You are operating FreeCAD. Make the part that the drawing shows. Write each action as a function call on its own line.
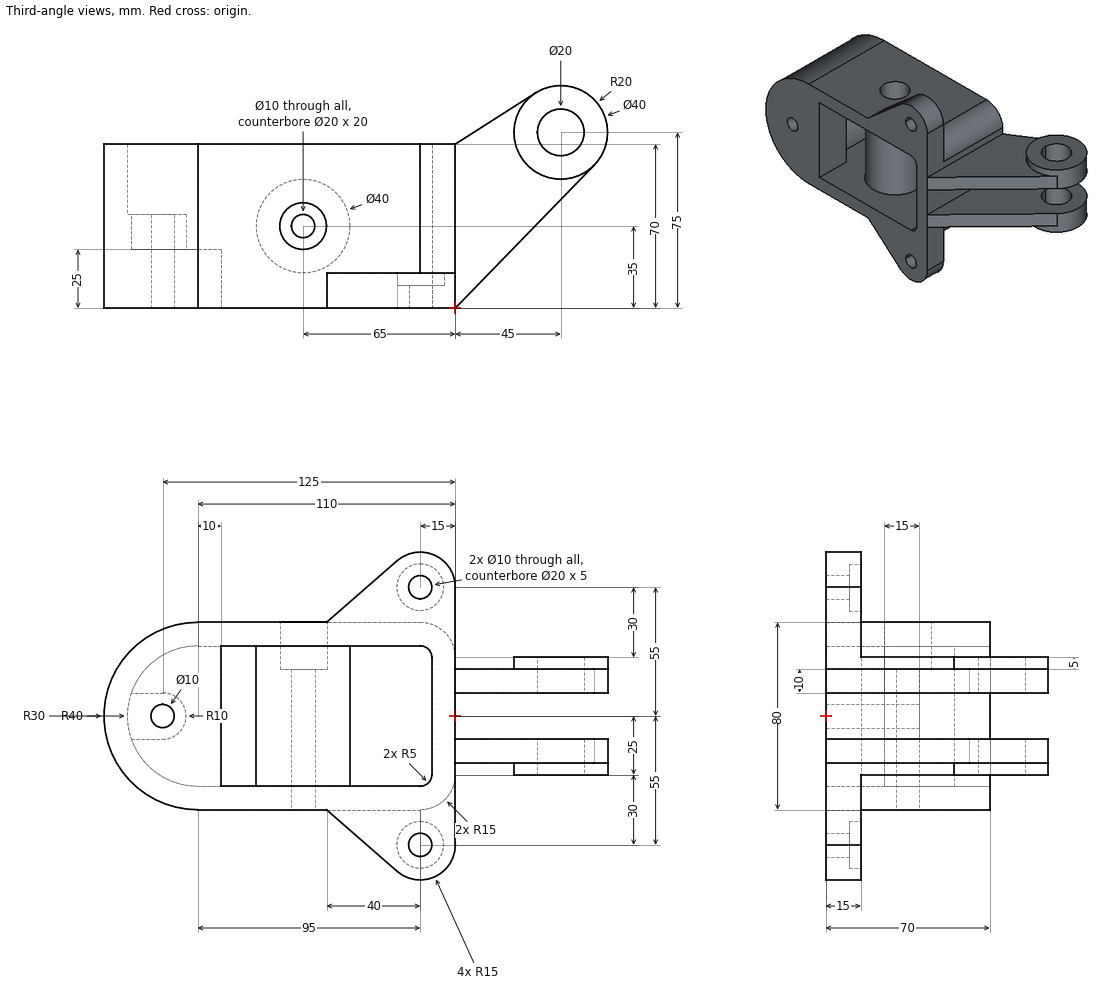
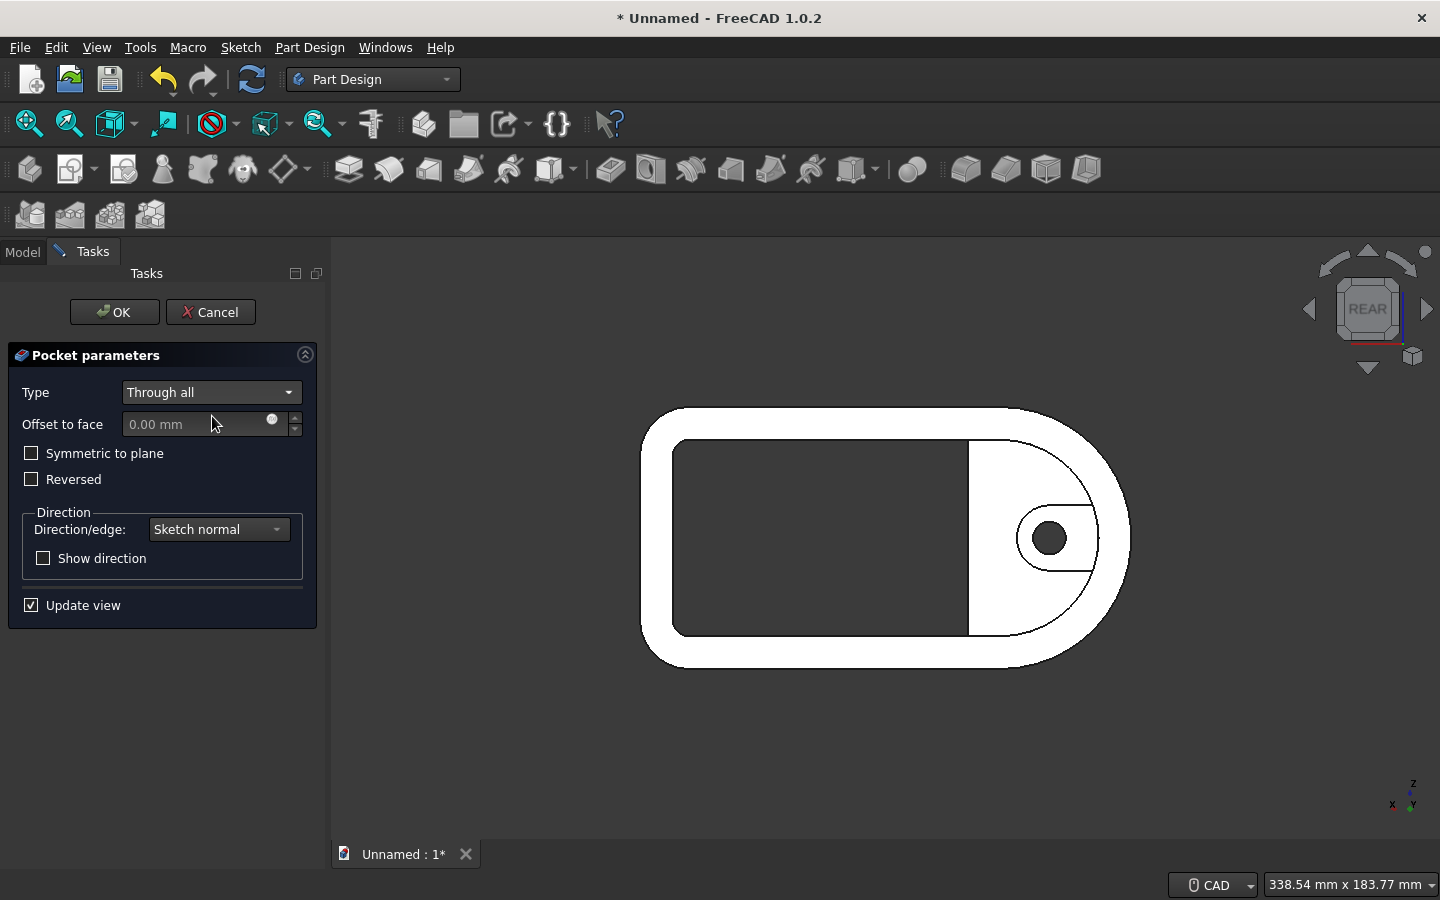
click(115, 312)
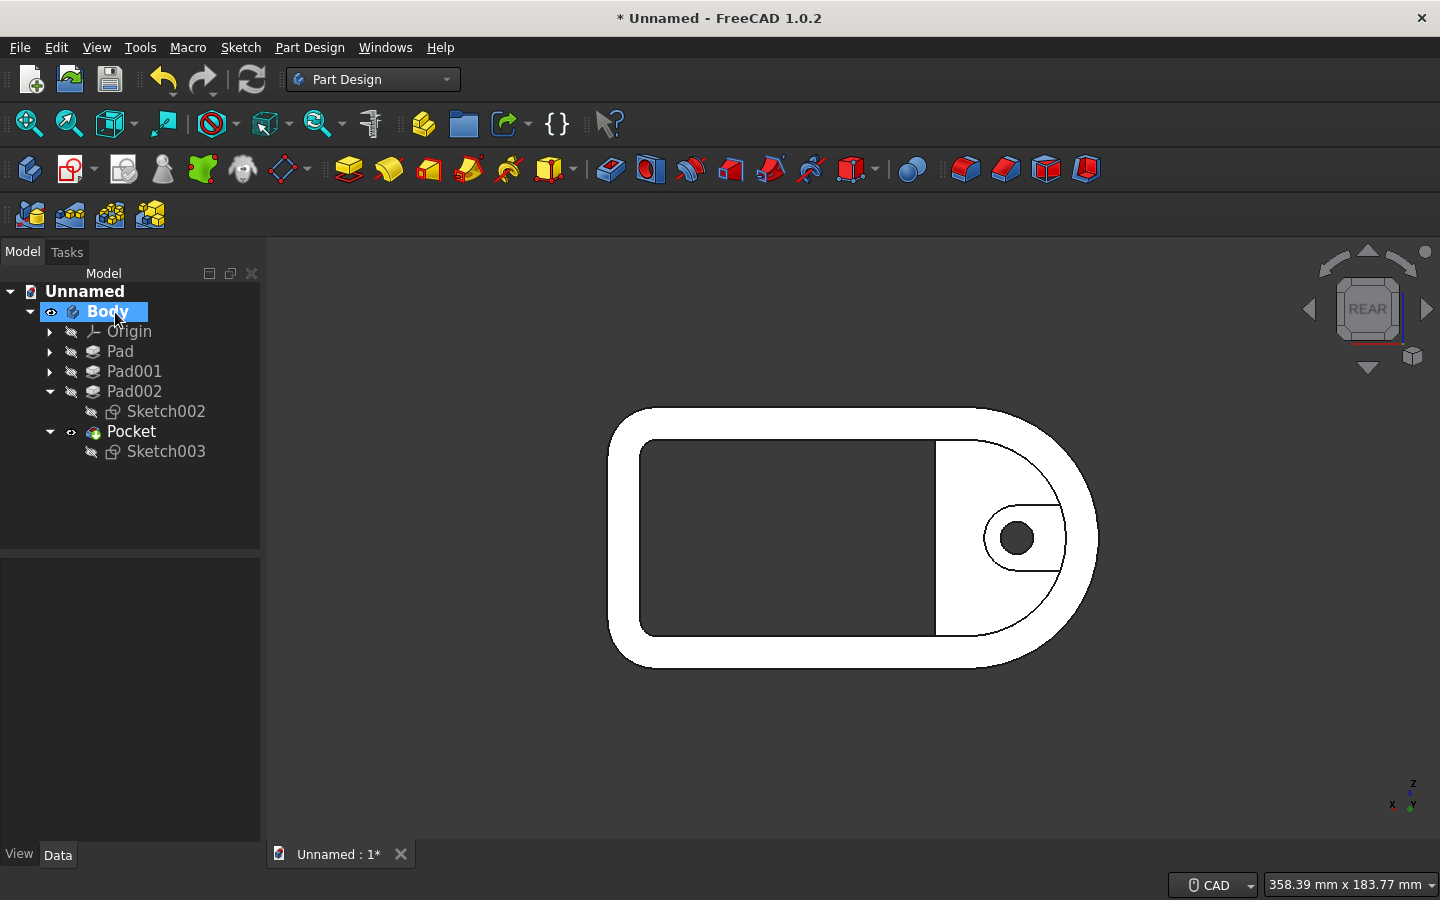
key(v)
key(f)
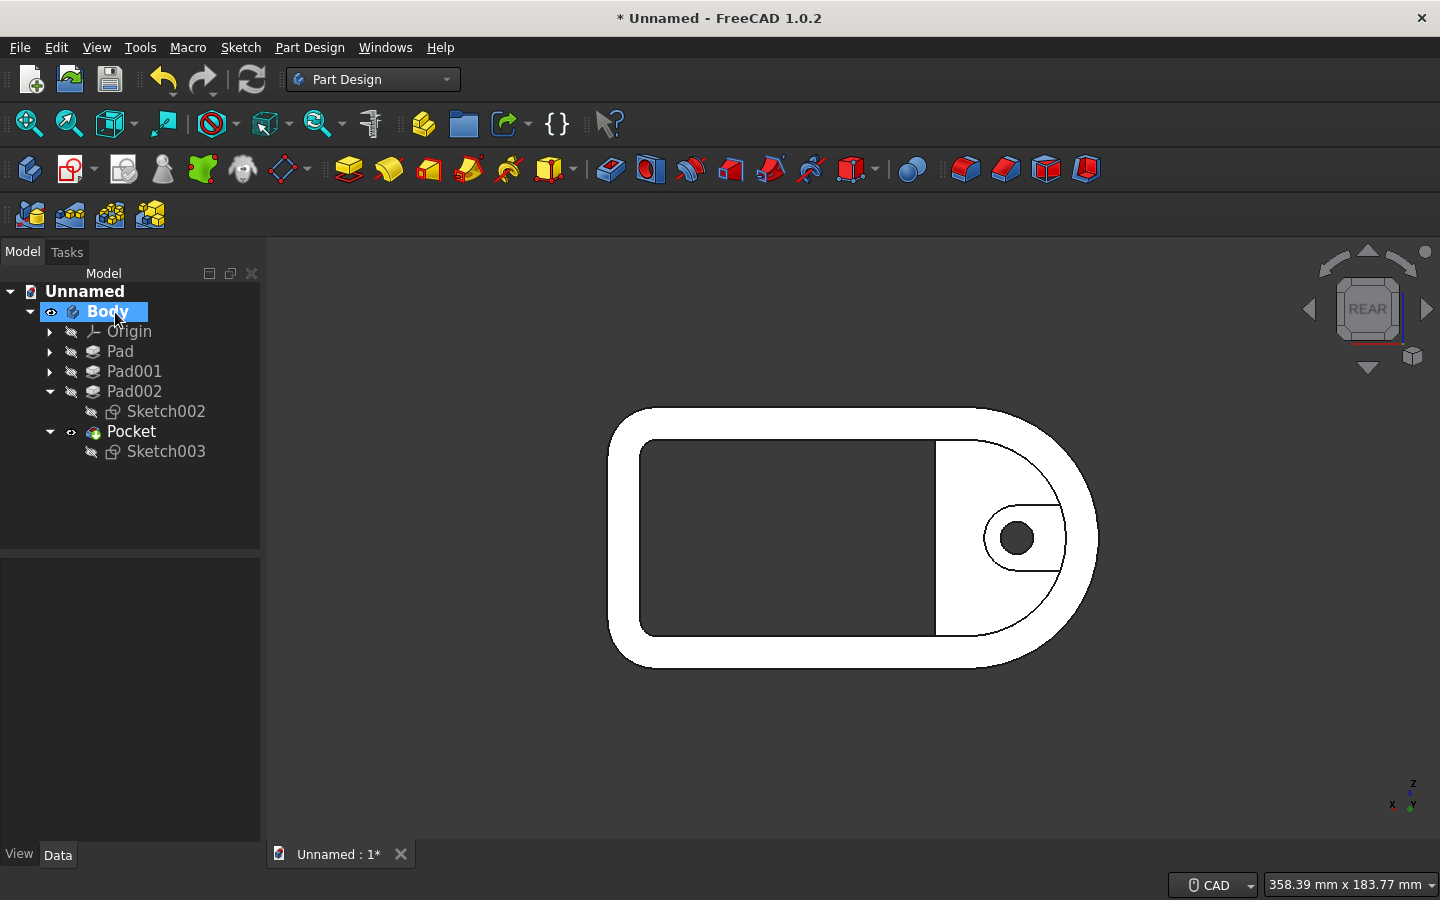
click(50, 332)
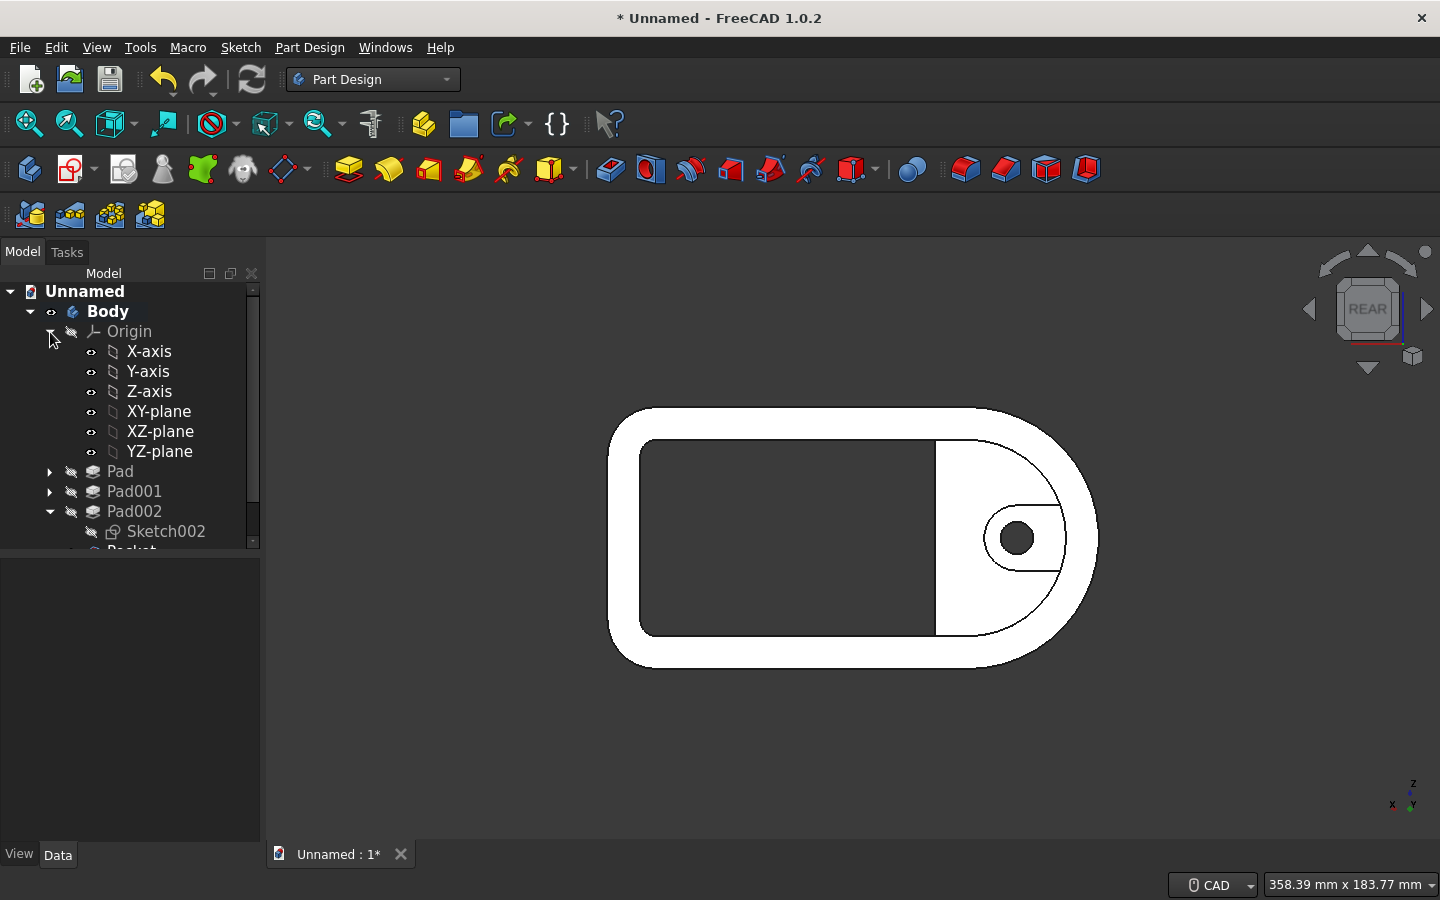
click(136, 412)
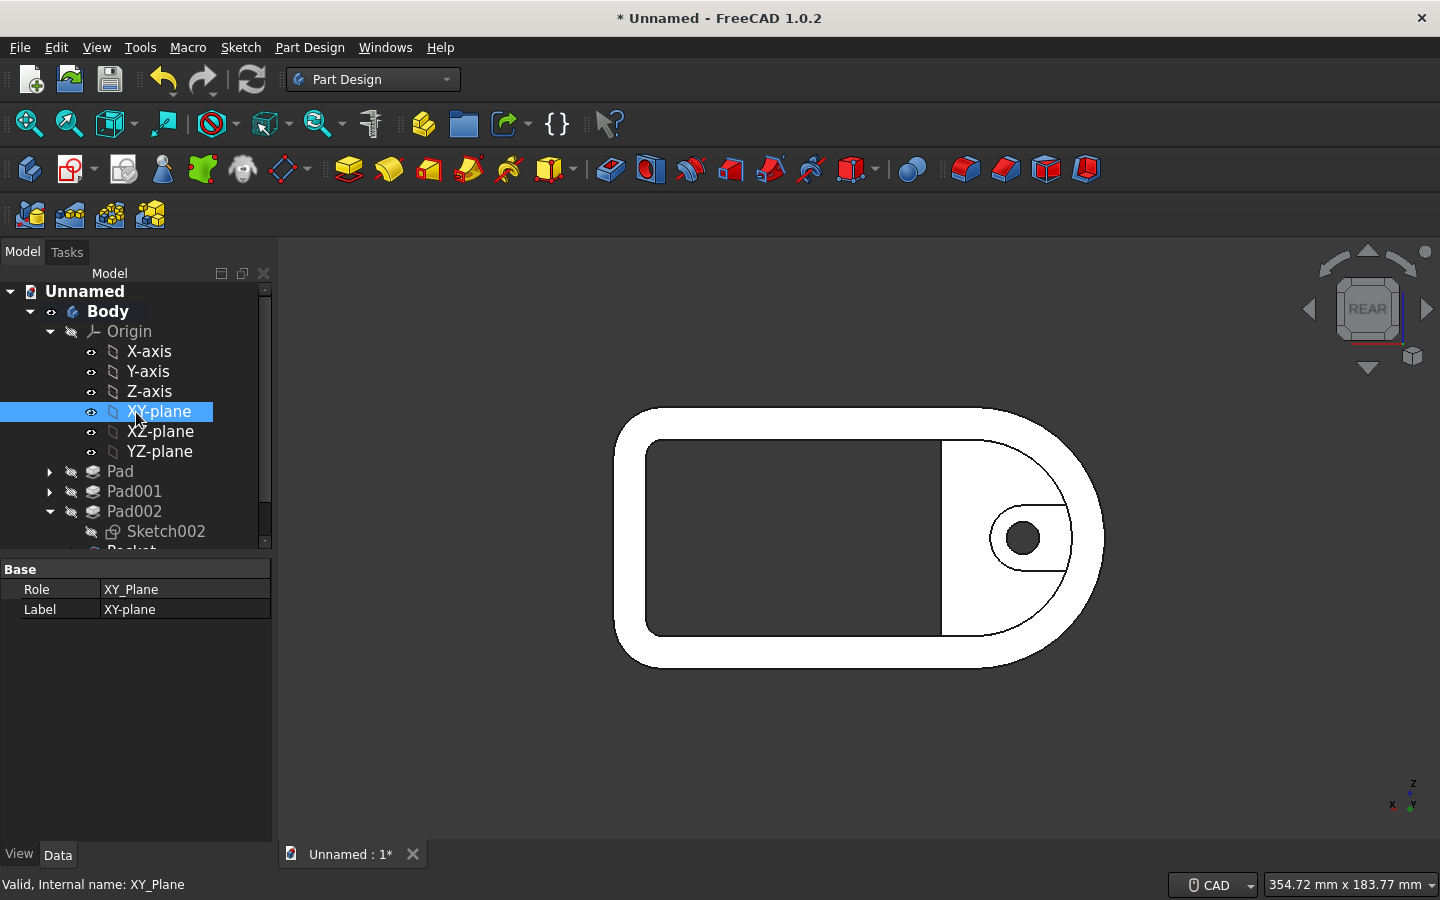
click(284, 170)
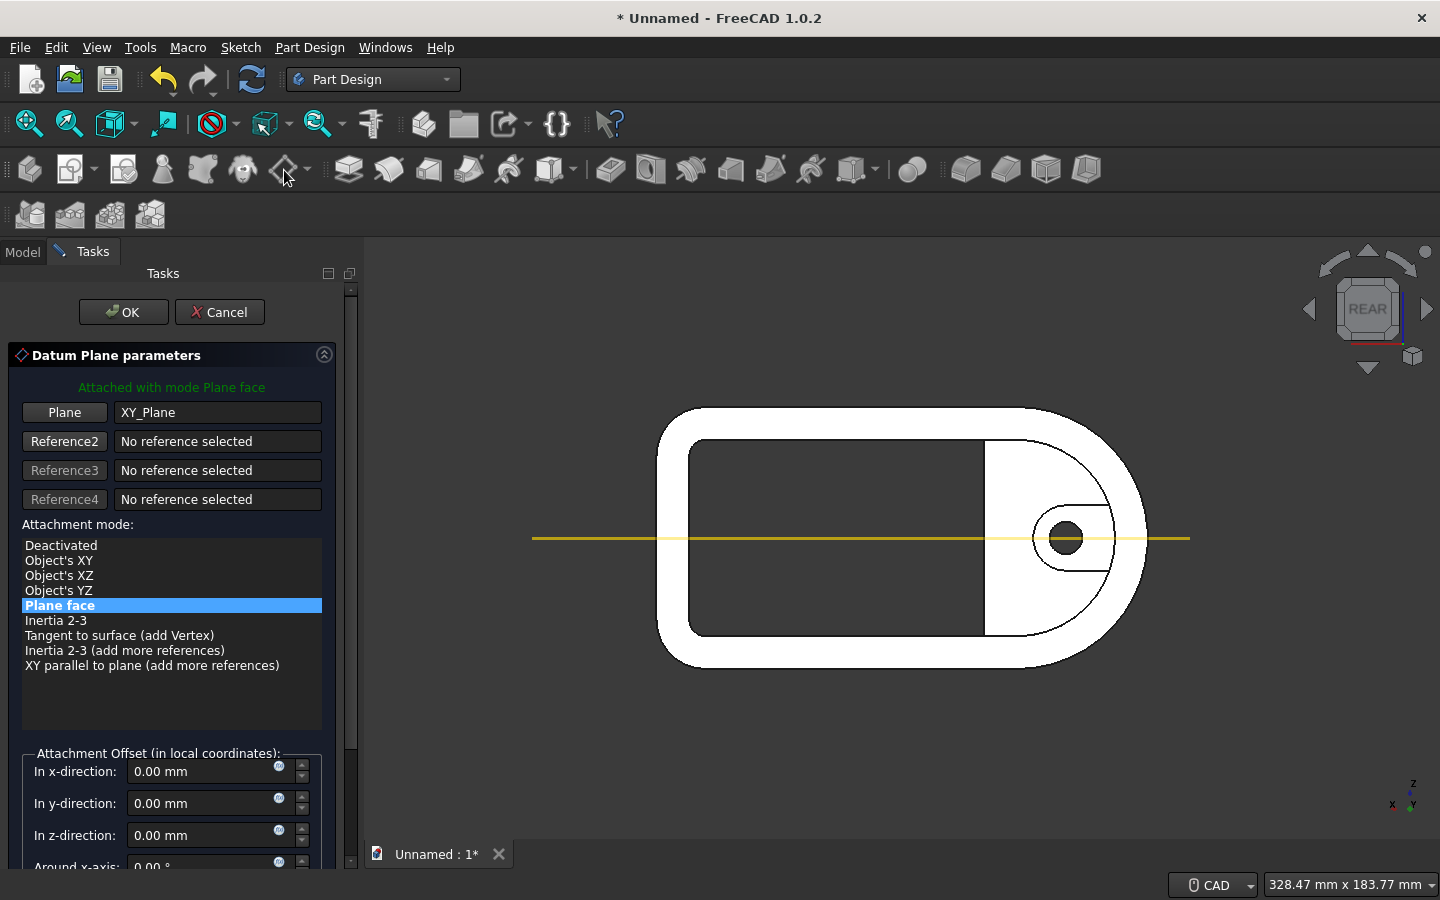
triple_click(210, 835)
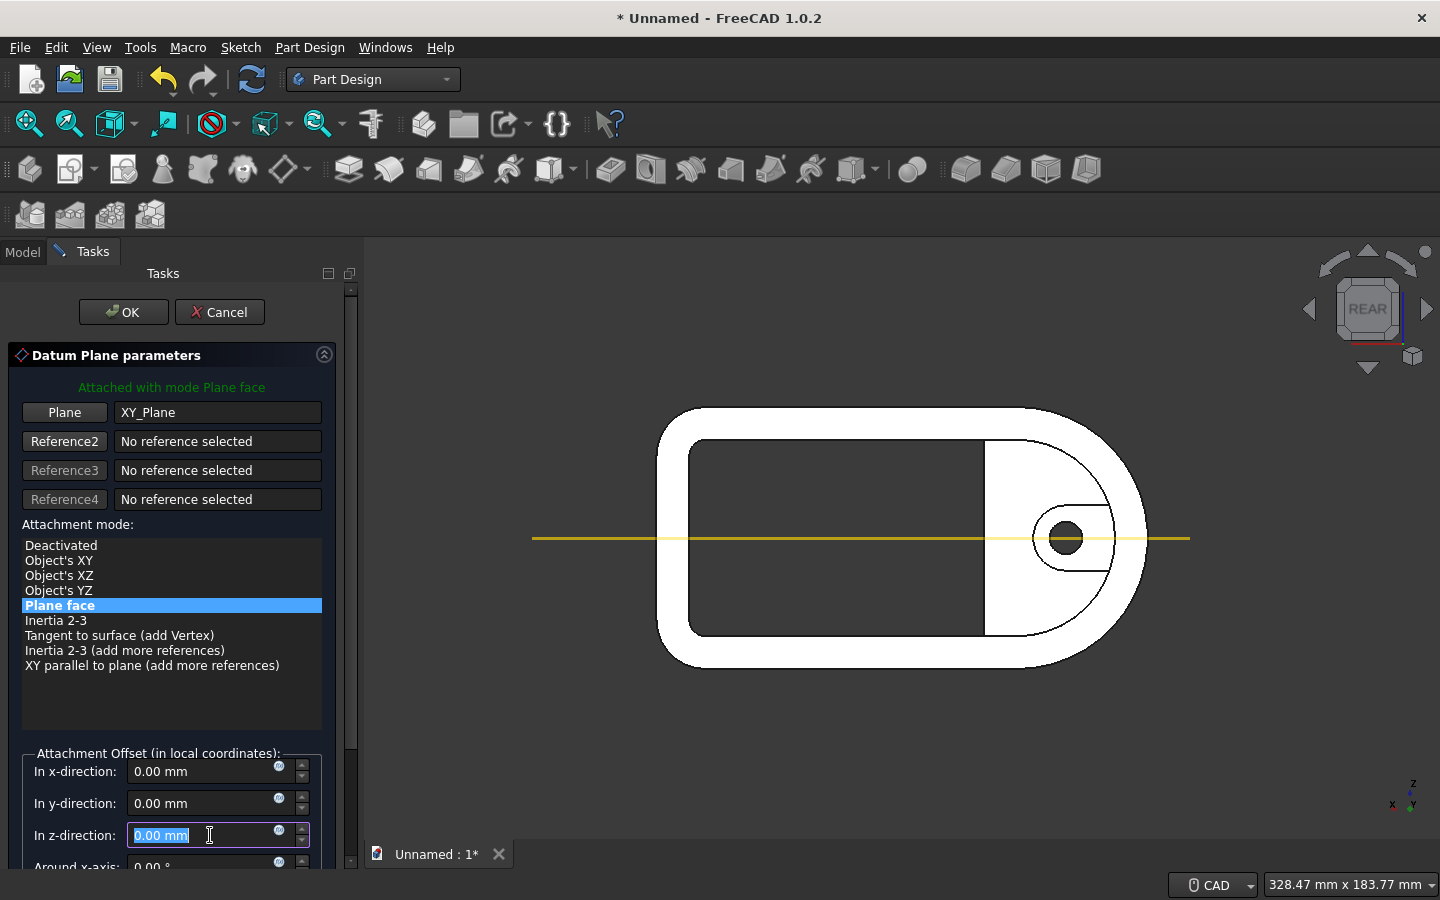
text(10)
key(Tab)